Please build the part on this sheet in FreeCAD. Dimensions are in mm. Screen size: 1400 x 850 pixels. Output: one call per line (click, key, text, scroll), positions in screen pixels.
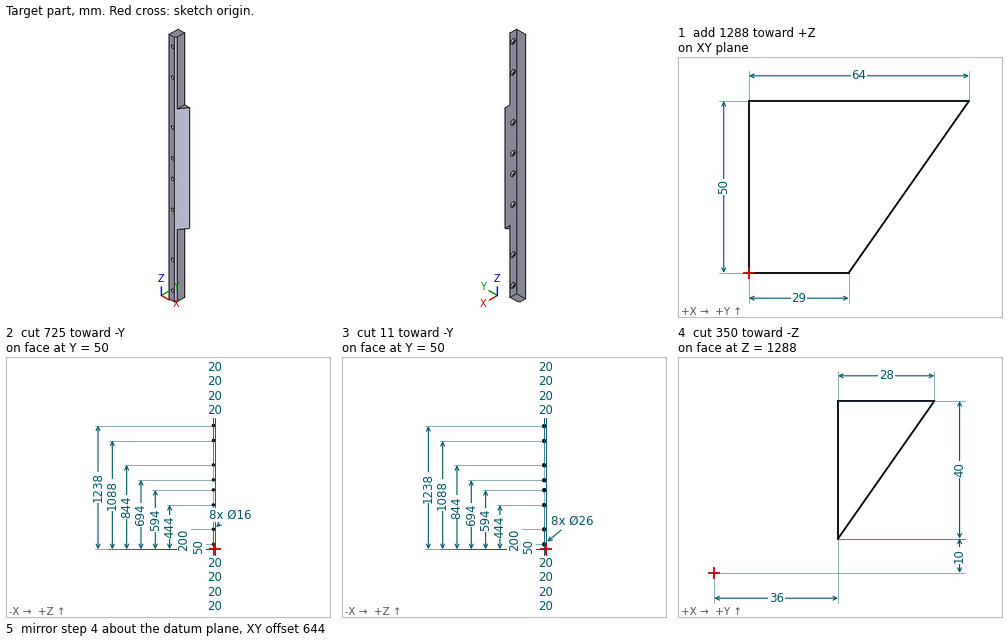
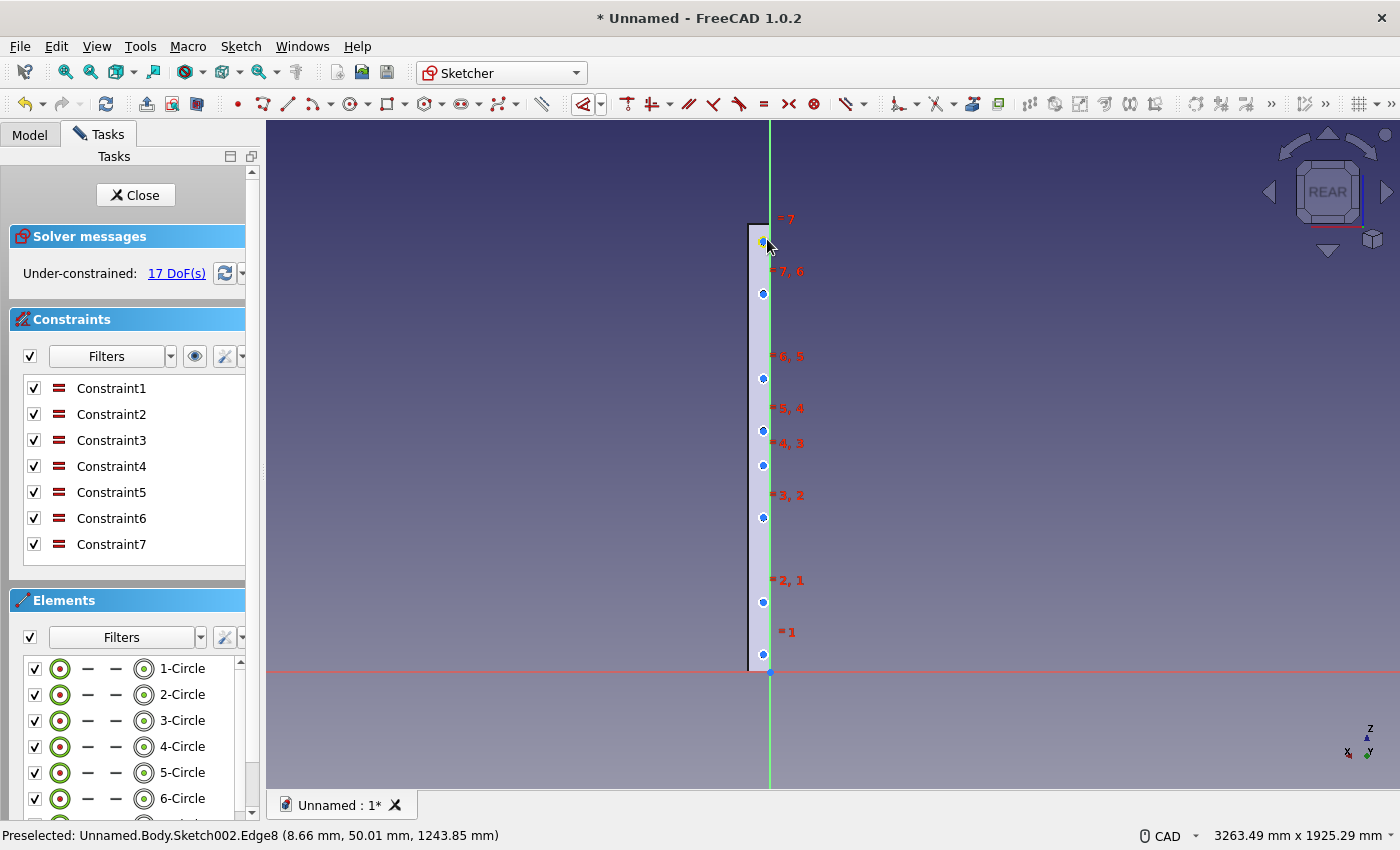
scroll(767, 652, up, 8)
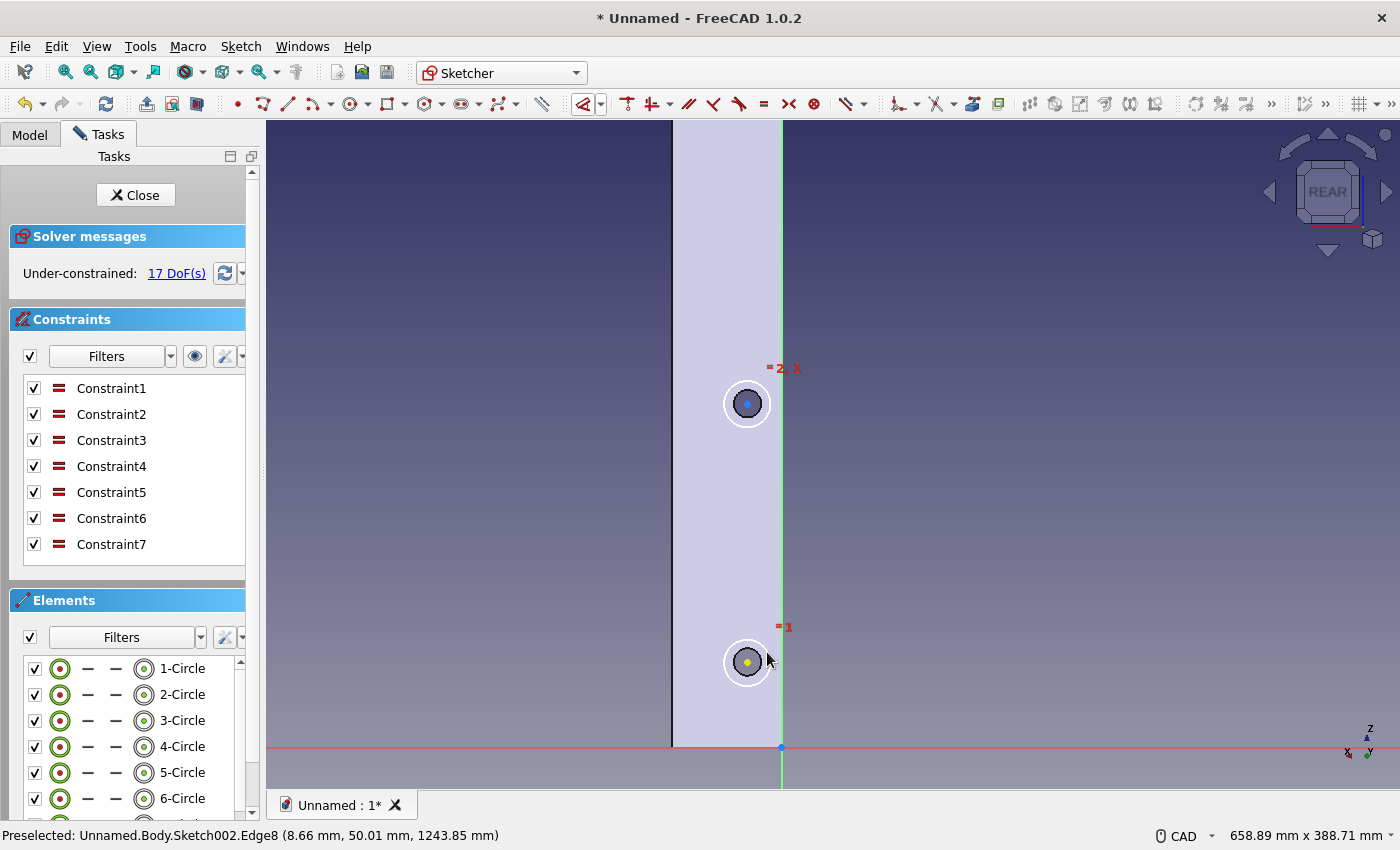
click(764, 647)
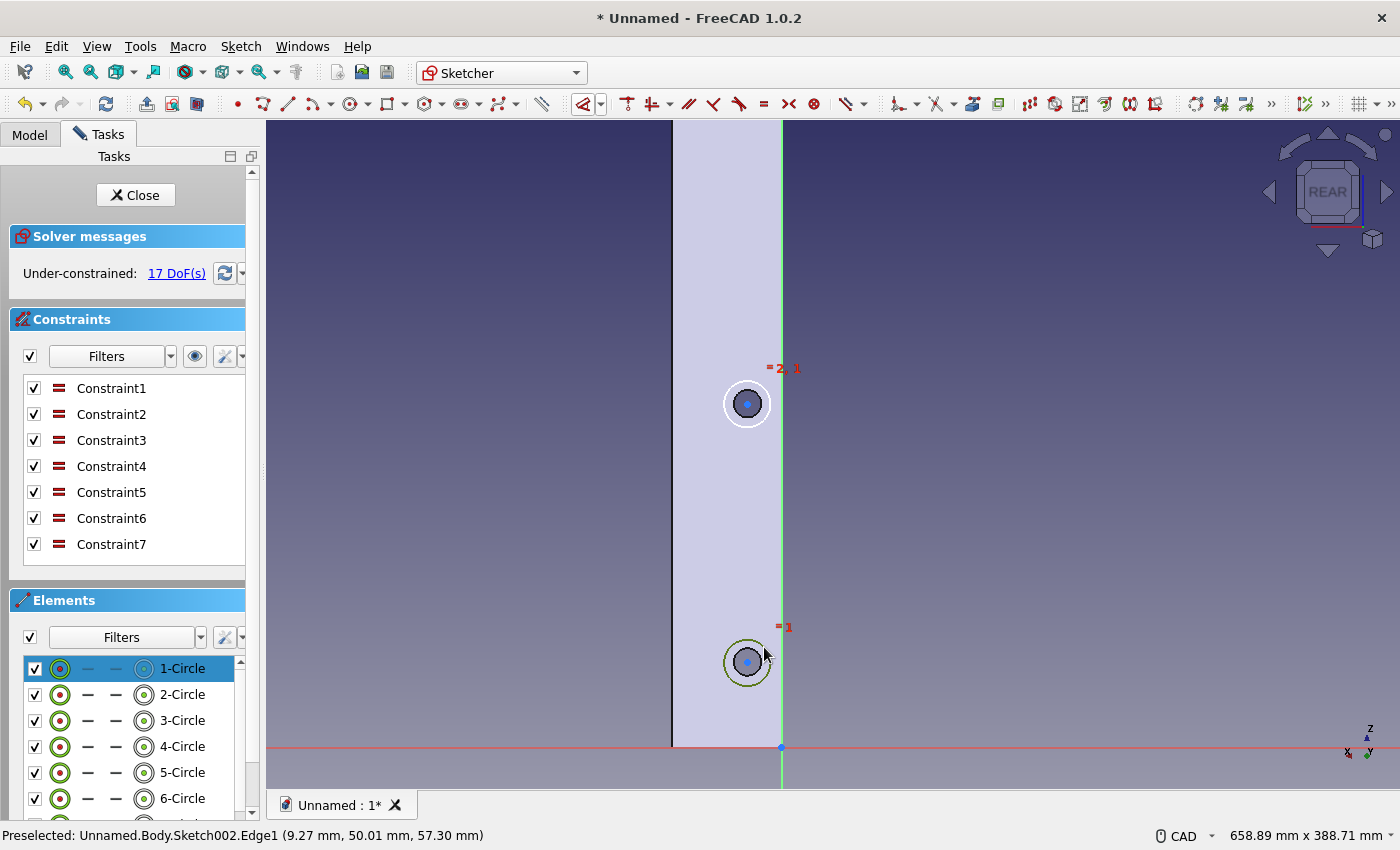
click(600, 104)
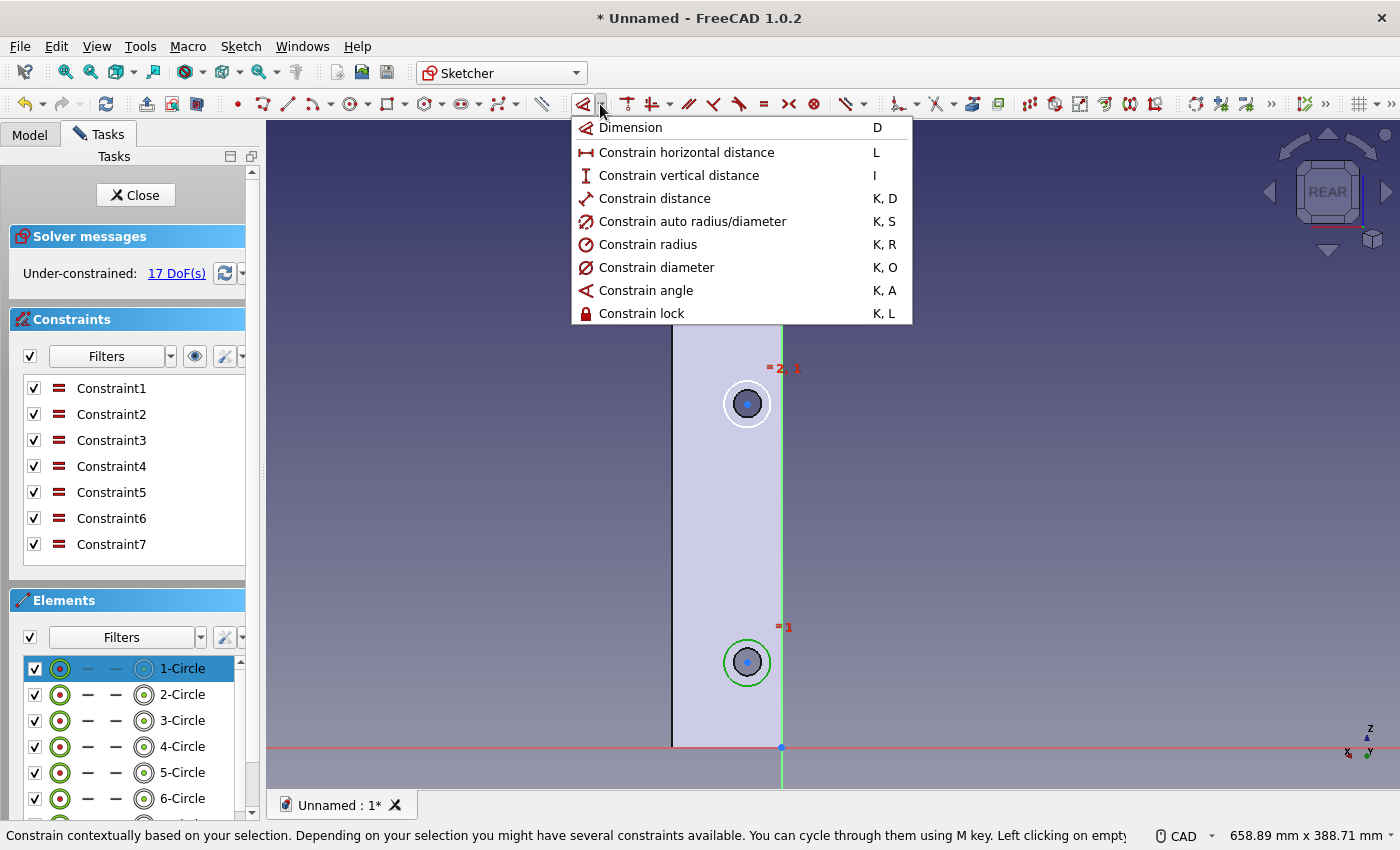
click(742, 268)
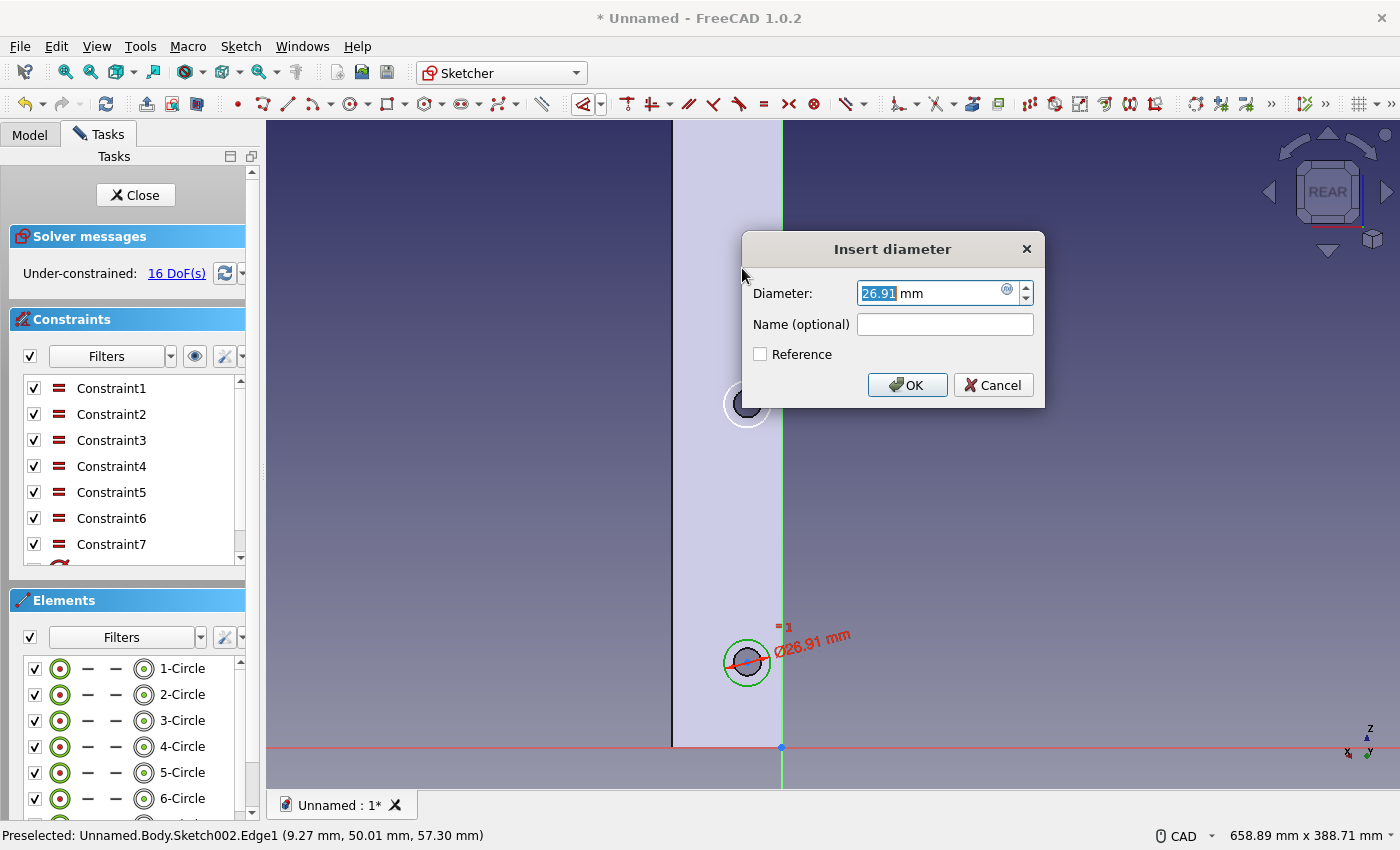
text(26)
key(Return)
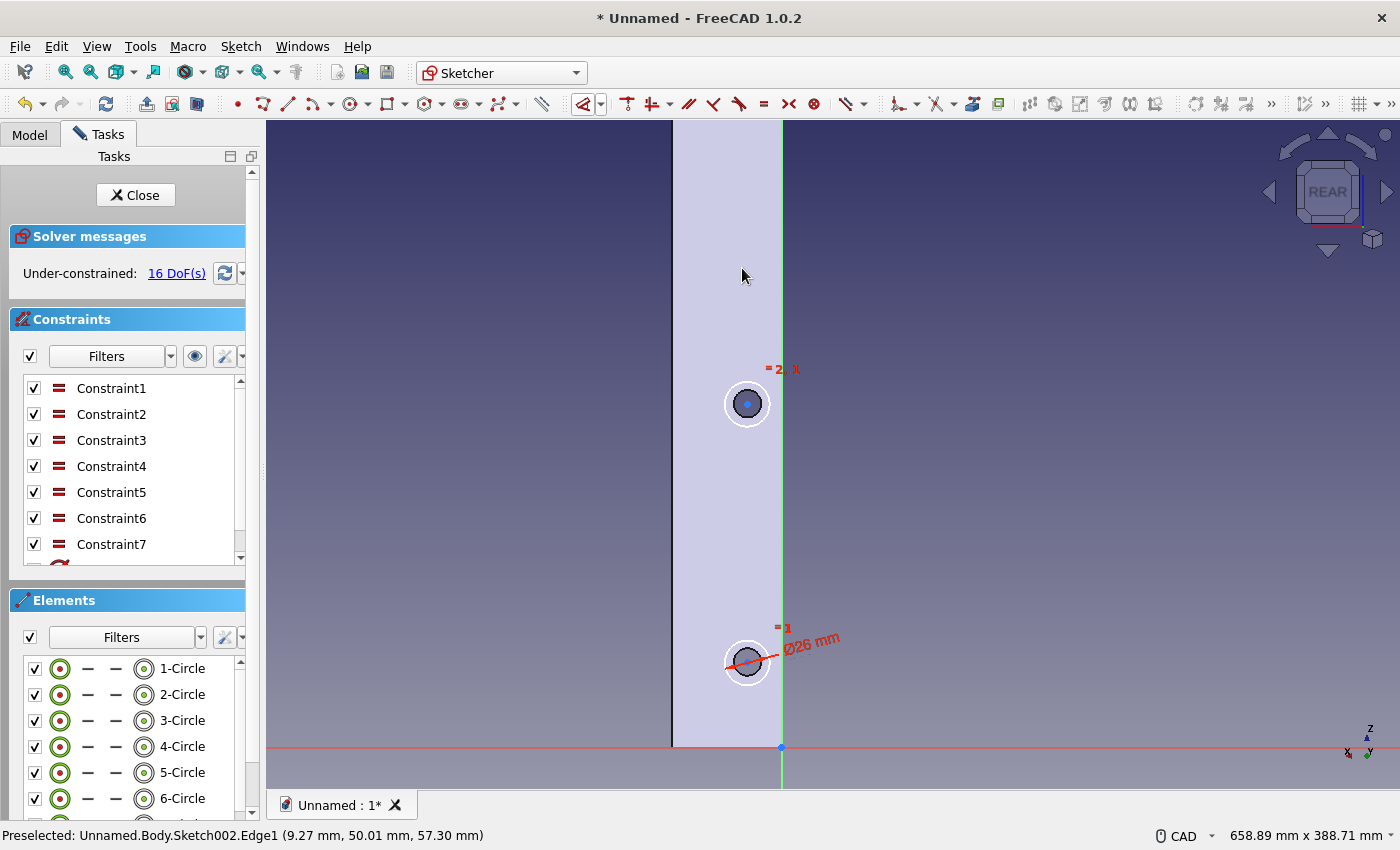
click(747, 663)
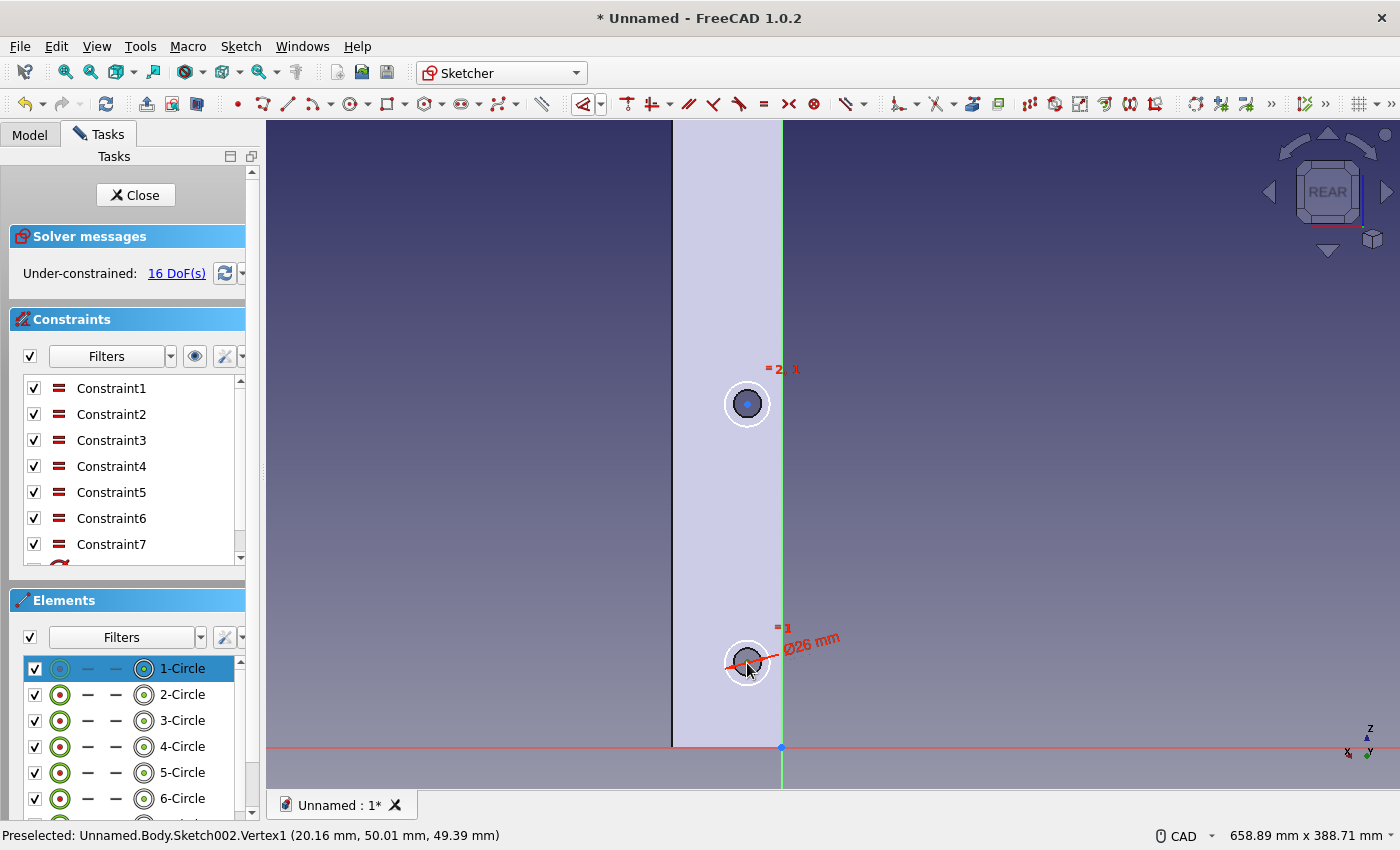
key(l)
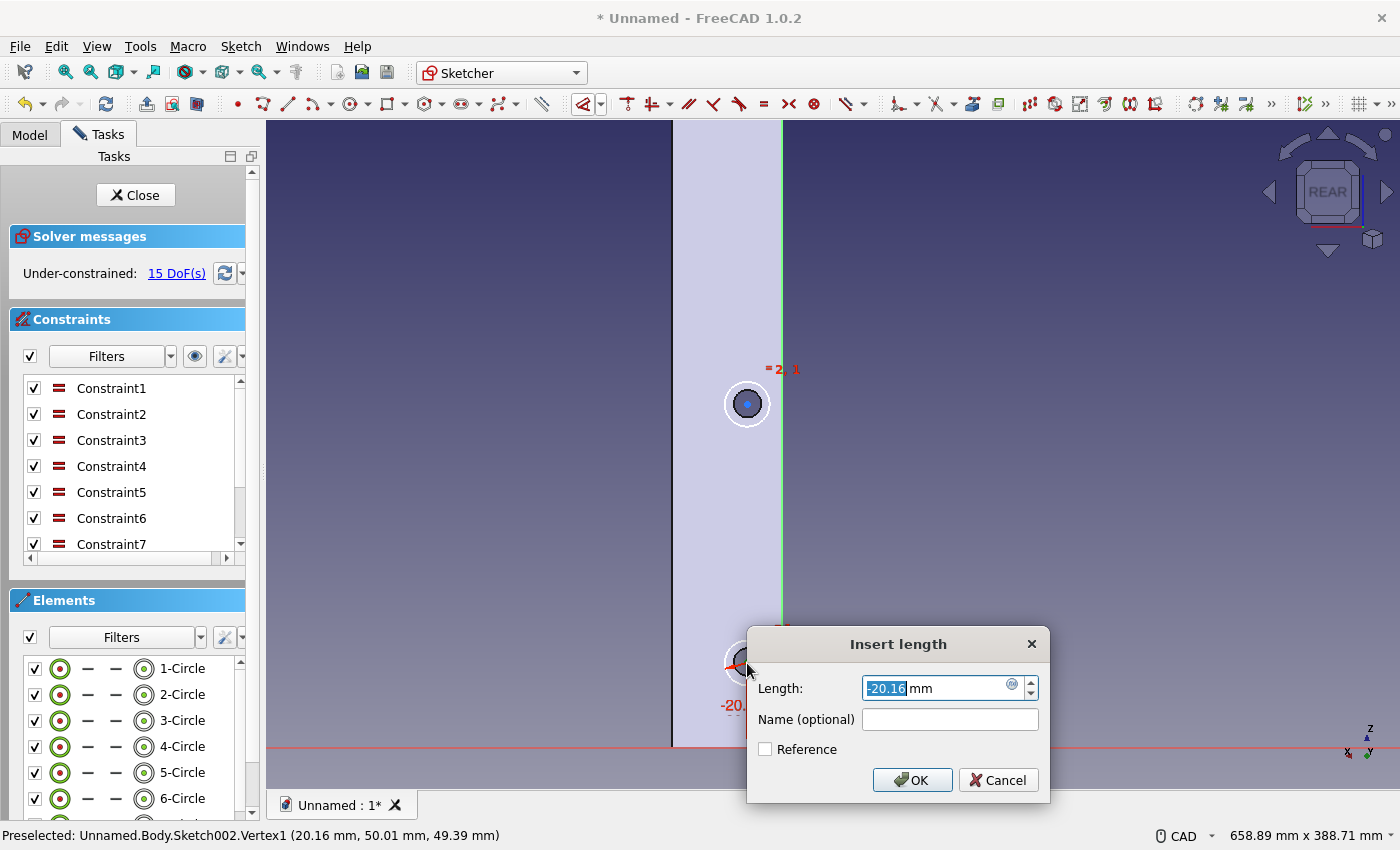
text(-20)
key(Return)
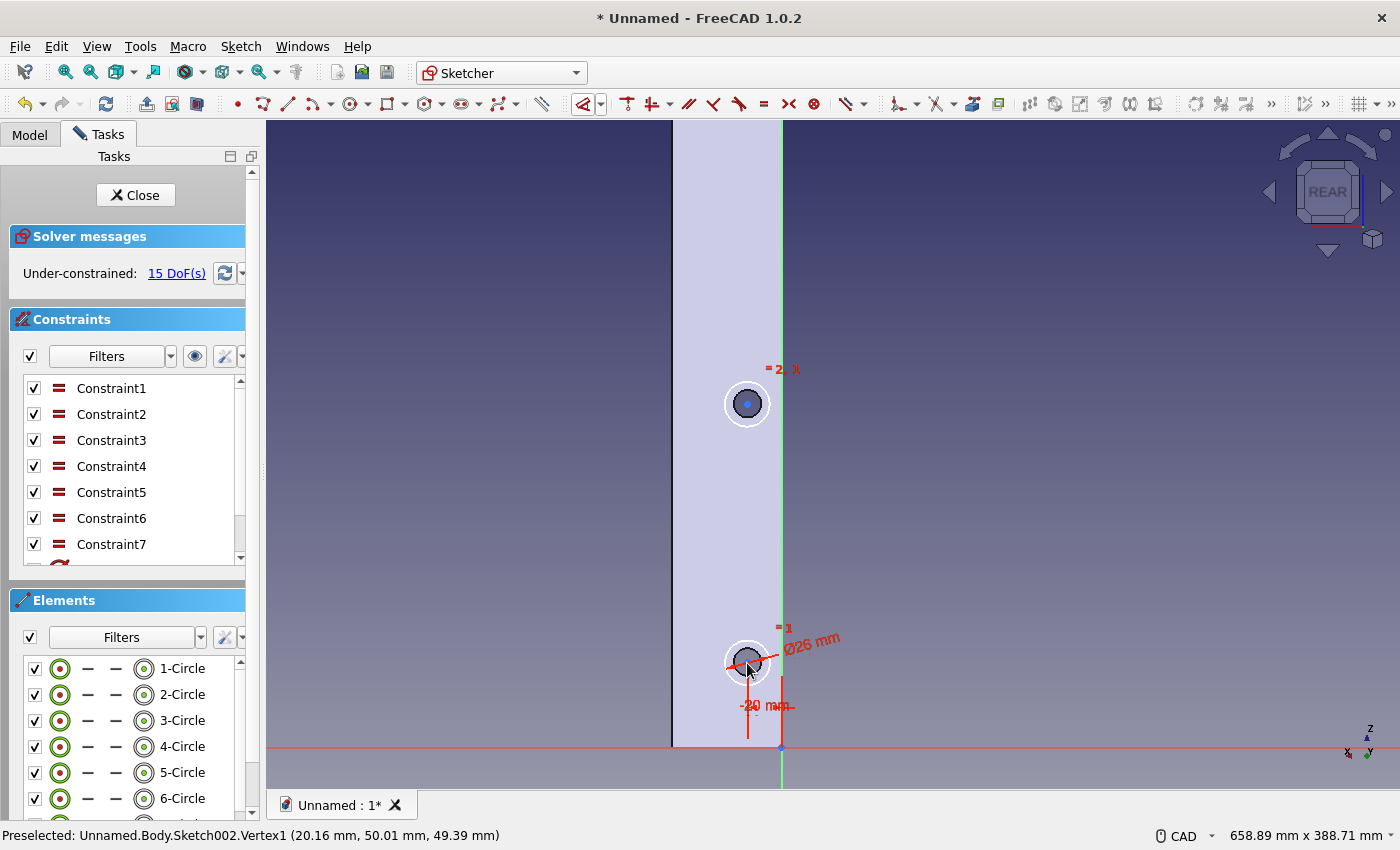
click(748, 663)